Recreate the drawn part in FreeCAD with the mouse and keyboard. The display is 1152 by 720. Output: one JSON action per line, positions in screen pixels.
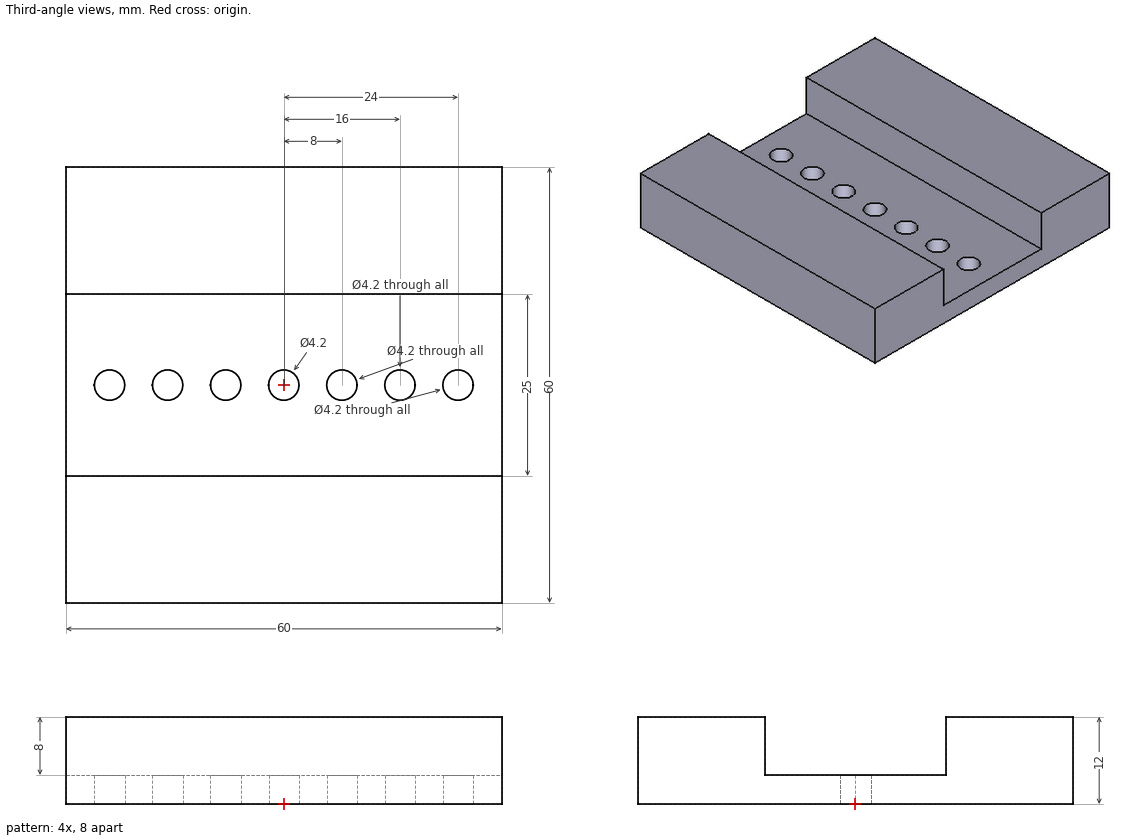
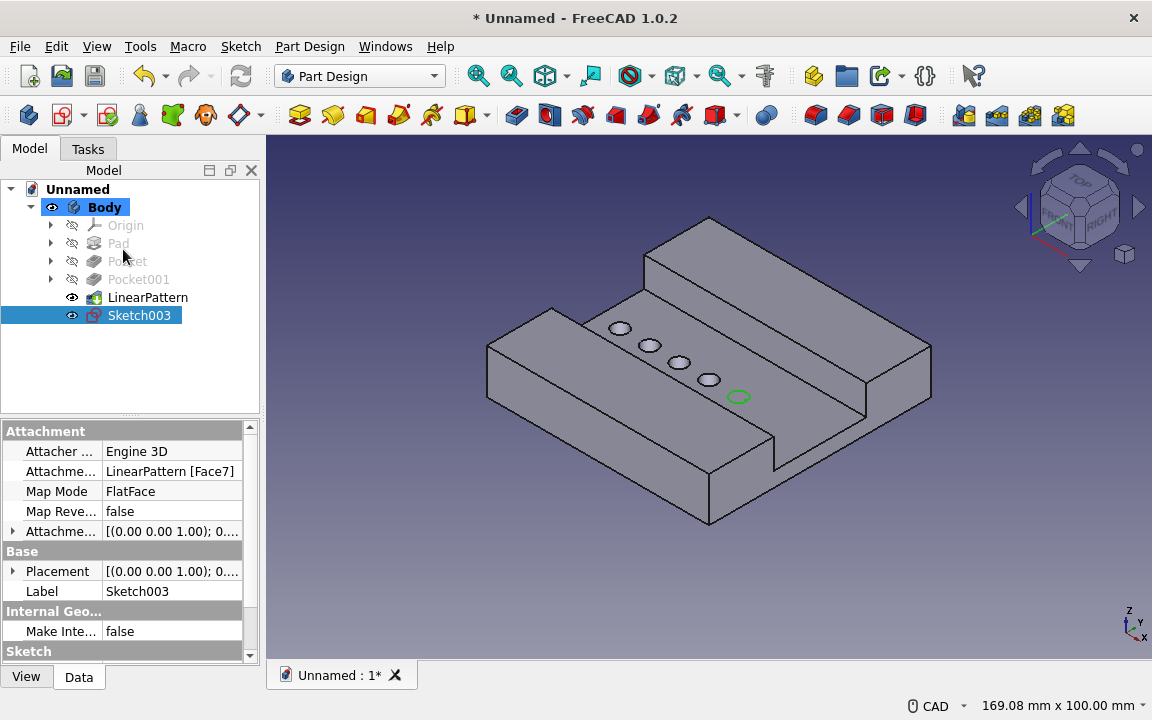
{"action": "left_click", "coordinate": [550, 116]}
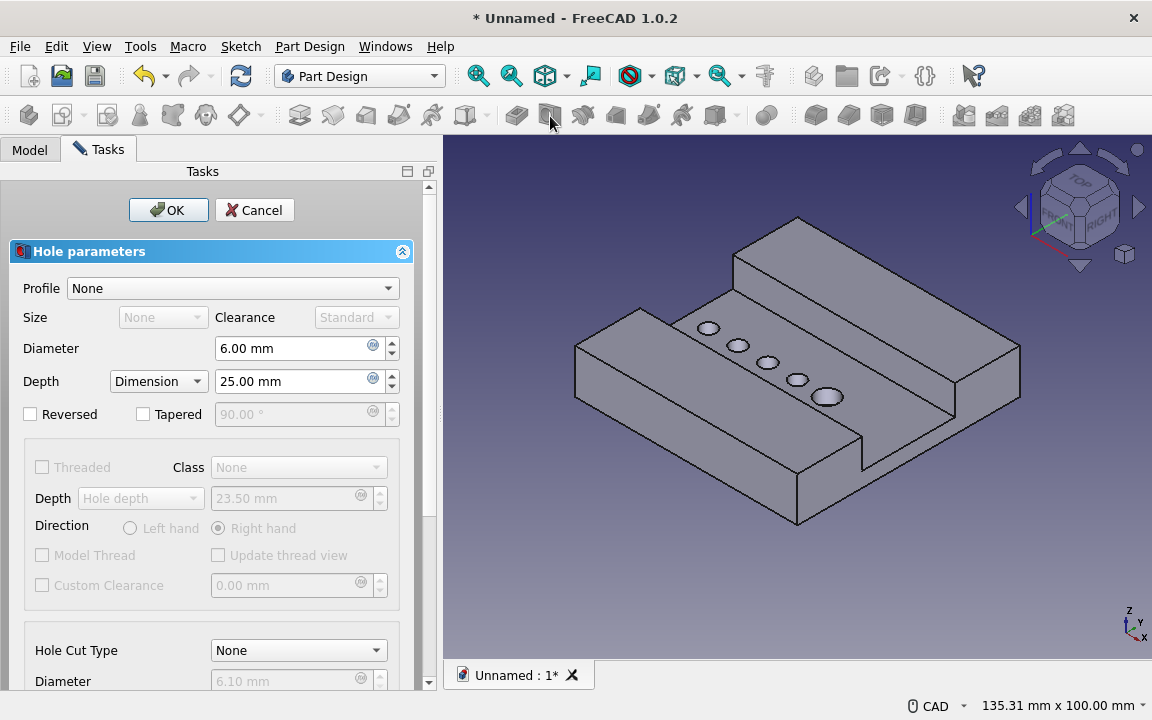
{"action": "triple_click", "coordinate": [300, 348]}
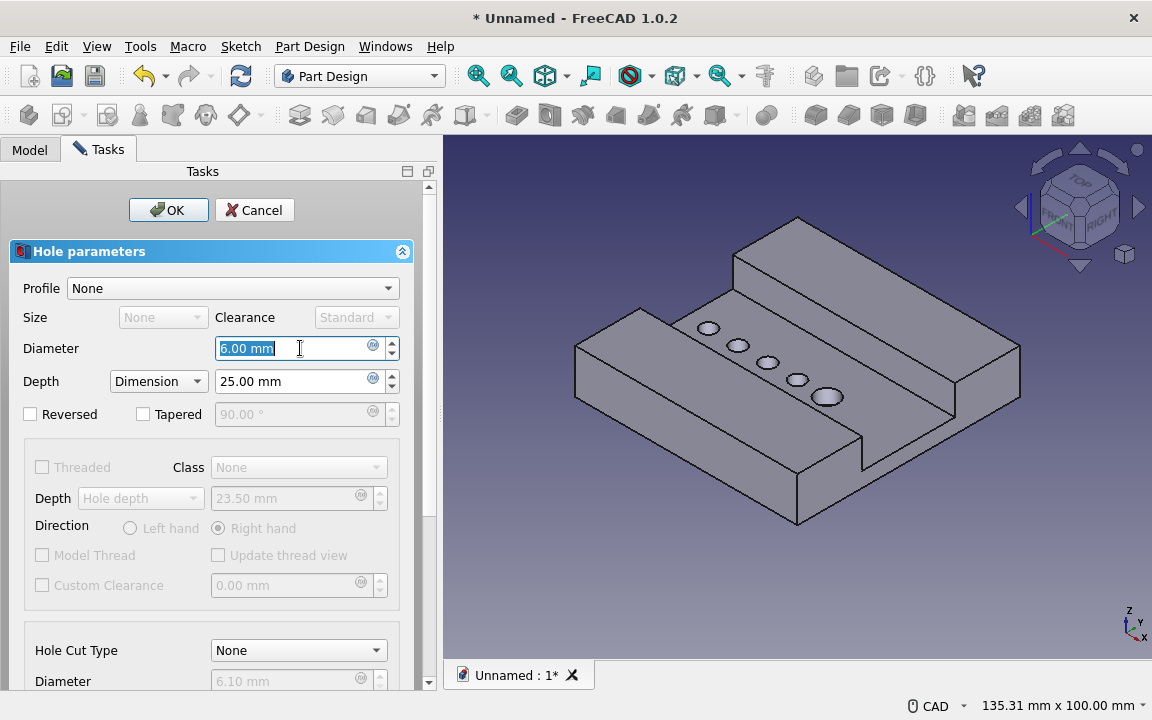
{"action": "type", "text": "4.2"}
{"action": "key", "text": "Tab"}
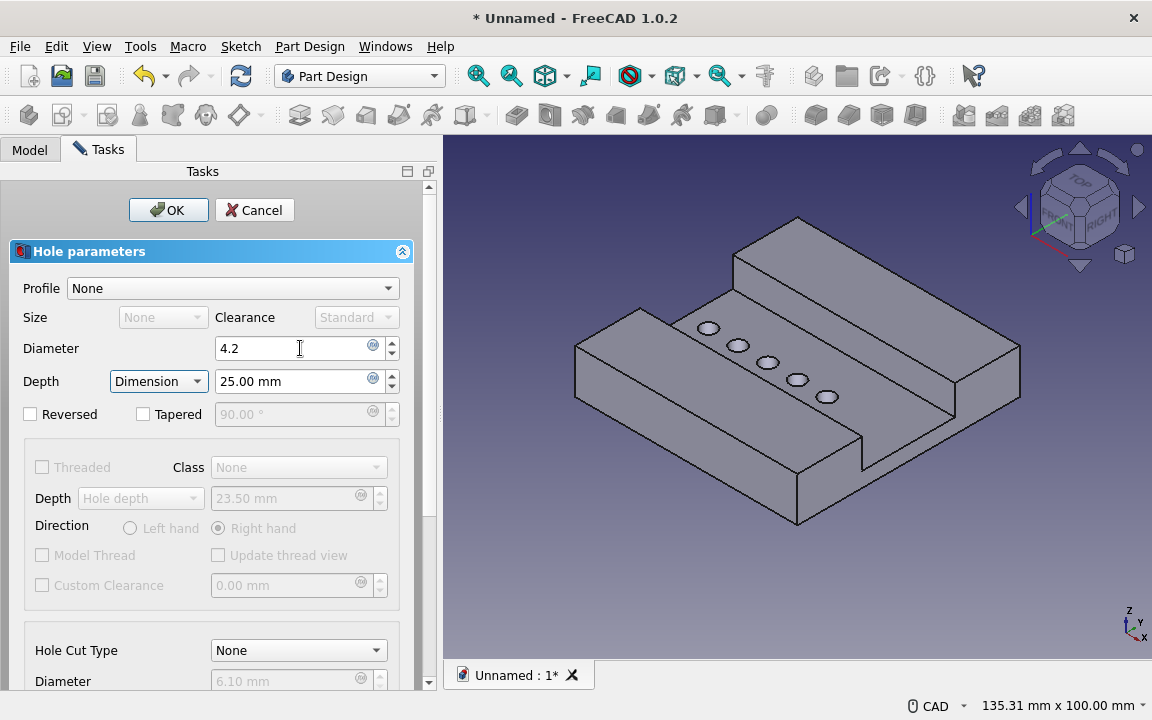
{"action": "left_click", "coordinate": [160, 382]}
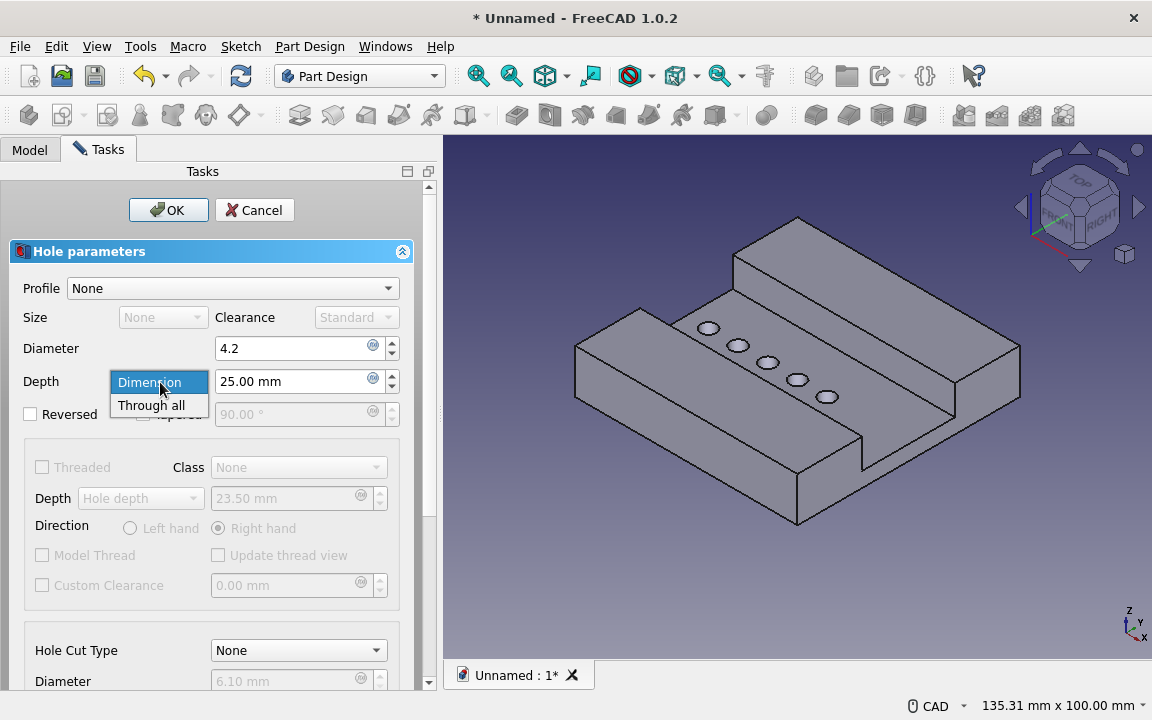
{"action": "left_click", "coordinate": [158, 406]}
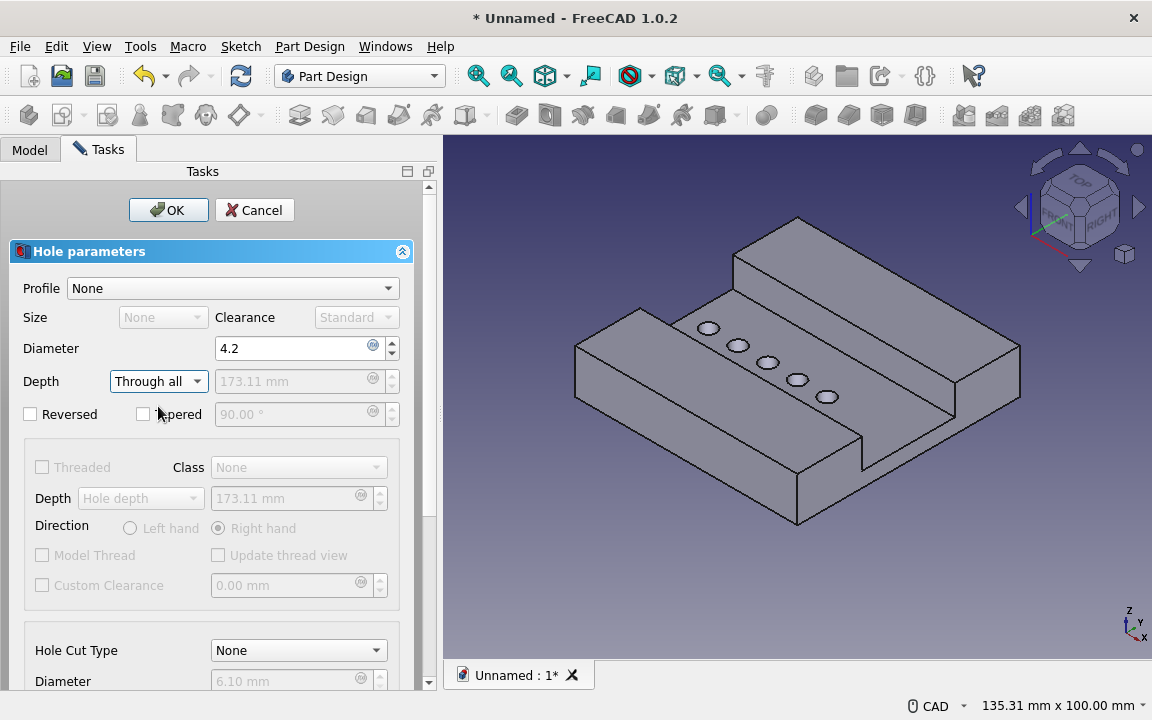
{"action": "left_click", "coordinate": [169, 210]}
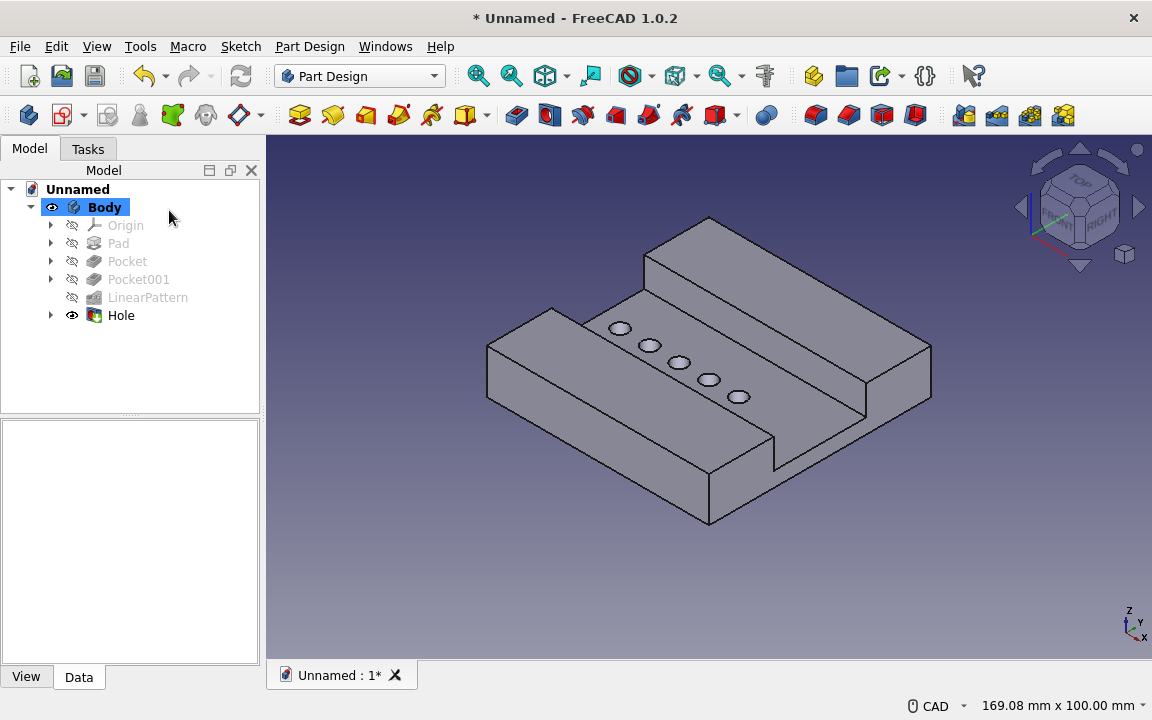
{"action": "left_click", "coordinate": [786, 408]}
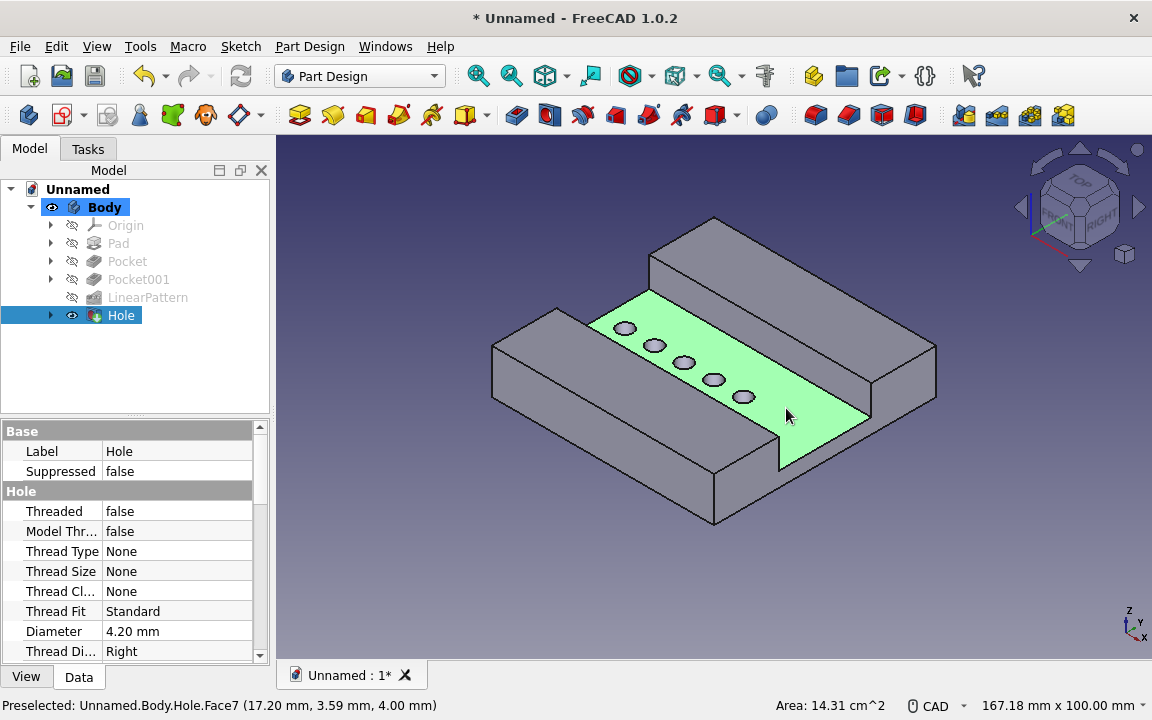
{"action": "left_click", "coordinate": [62, 116]}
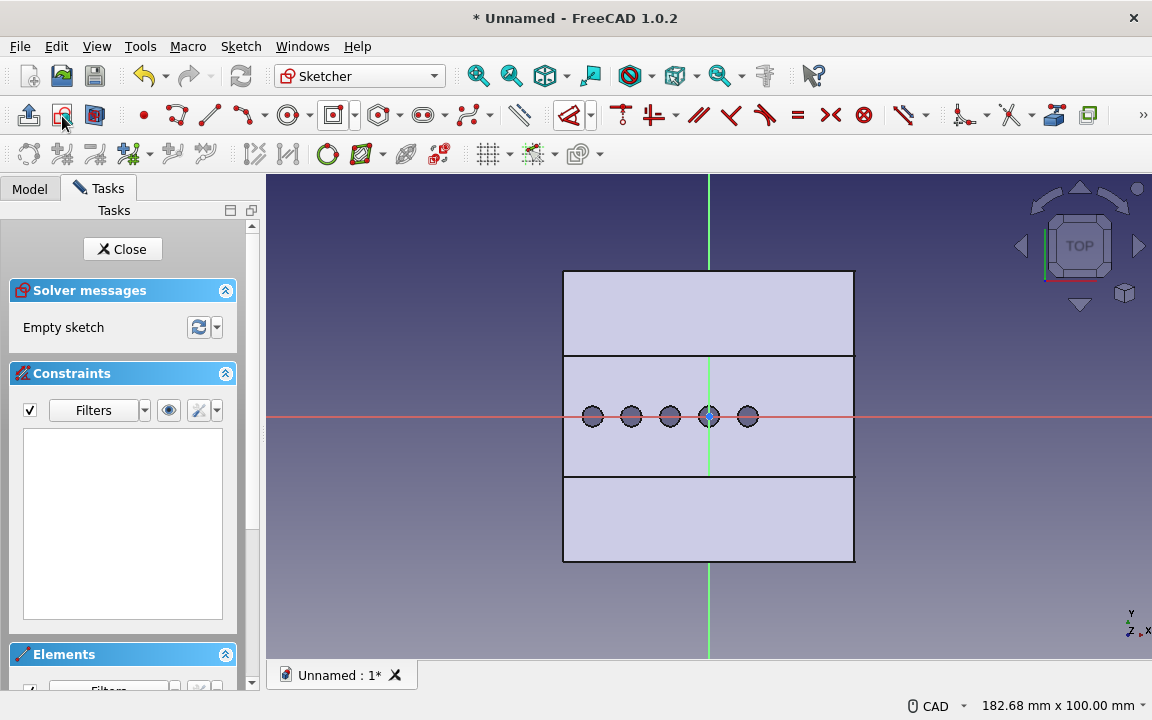
{"action": "left_click", "coordinate": [95, 116]}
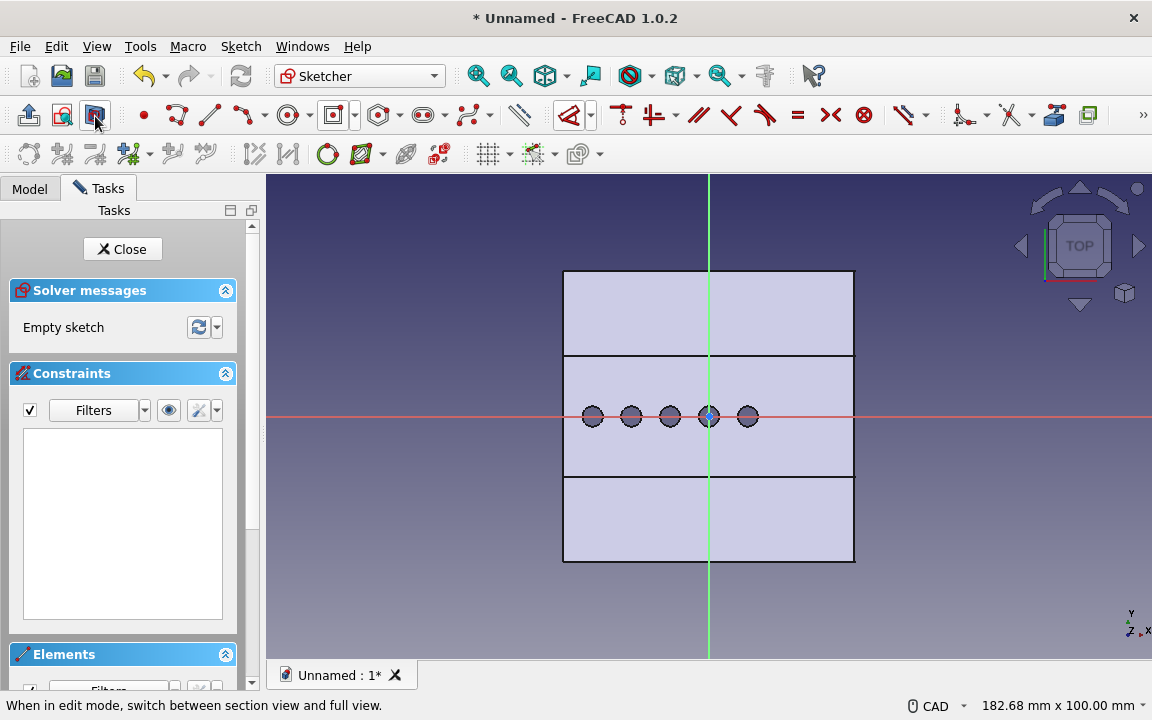
{"action": "scroll", "coordinate": [798, 416], "scroll_direction": "up", "scroll_amount": 13}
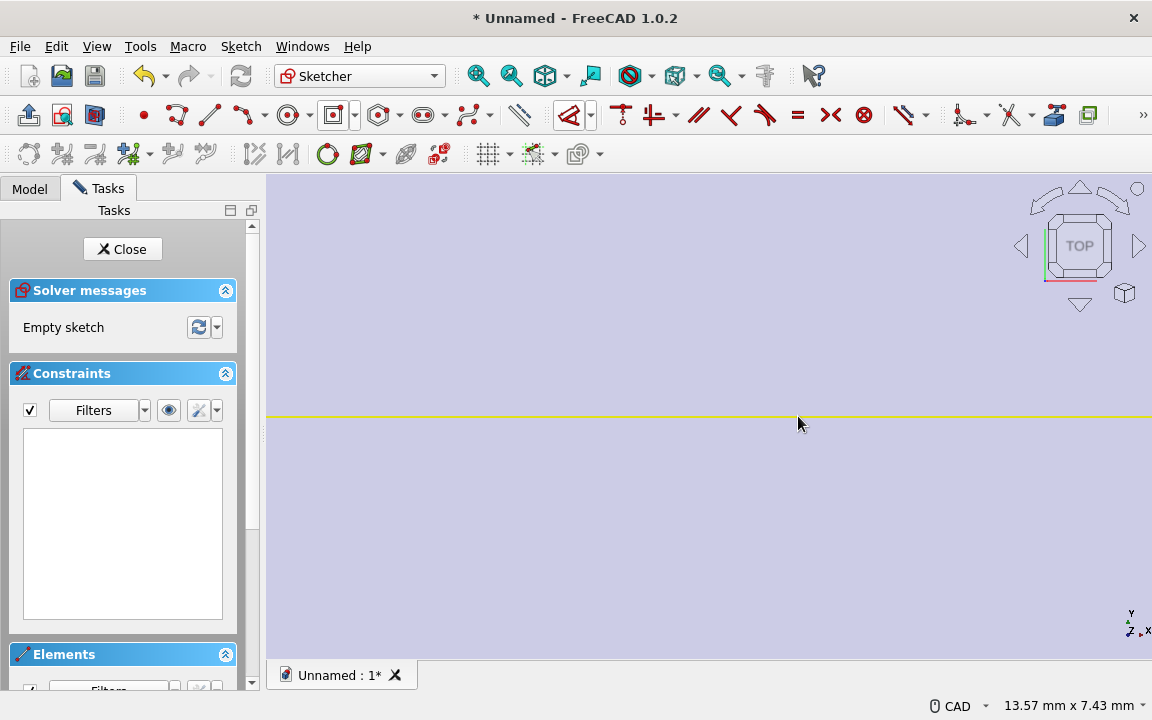
{"action": "left_click", "coordinate": [288, 116]}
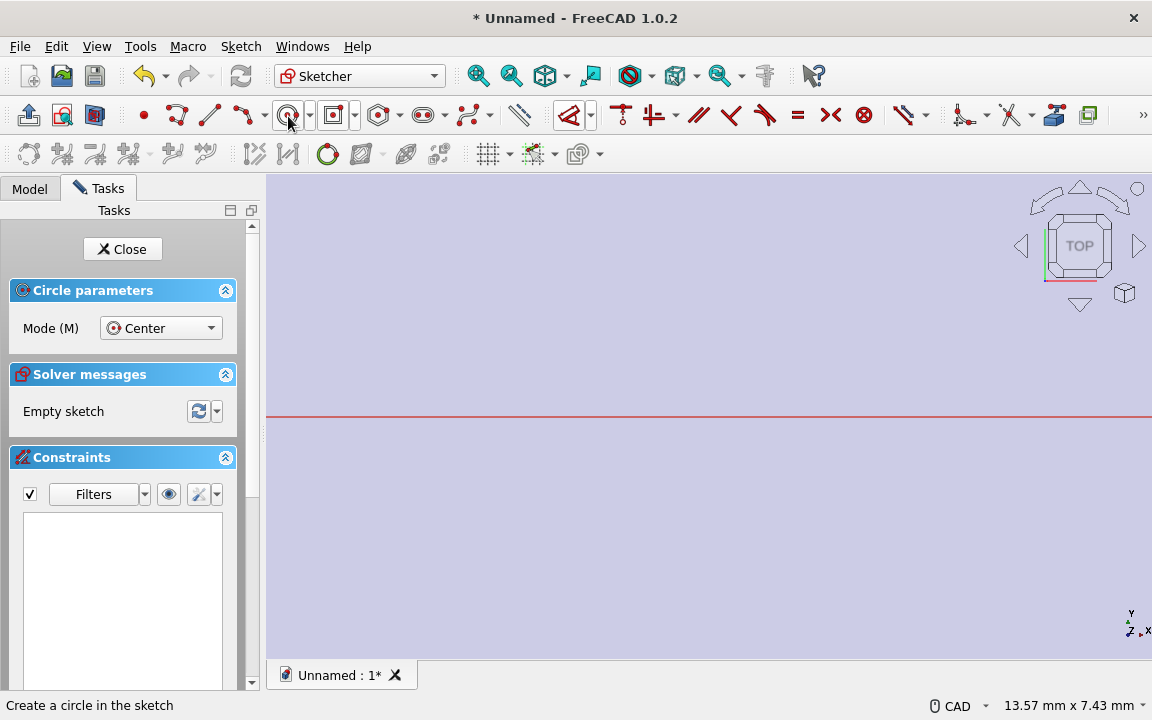
{"action": "left_click", "coordinate": [637, 416]}
{"action": "mouse_move", "coordinate": [734, 320]}